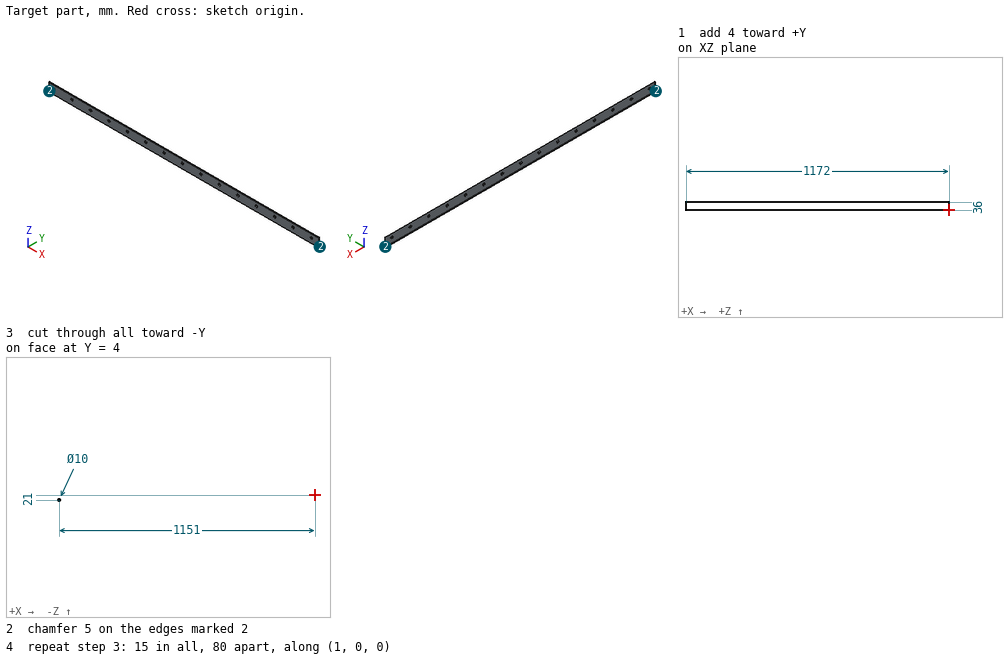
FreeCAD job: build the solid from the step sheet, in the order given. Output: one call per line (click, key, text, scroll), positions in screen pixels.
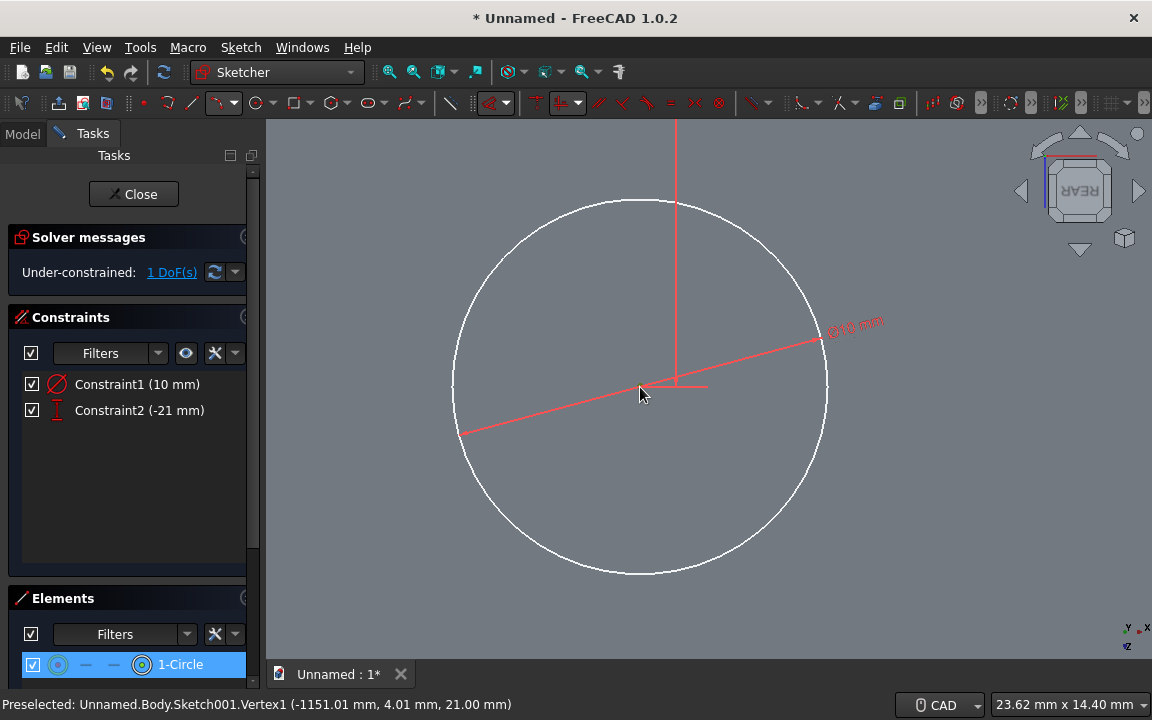
key(l)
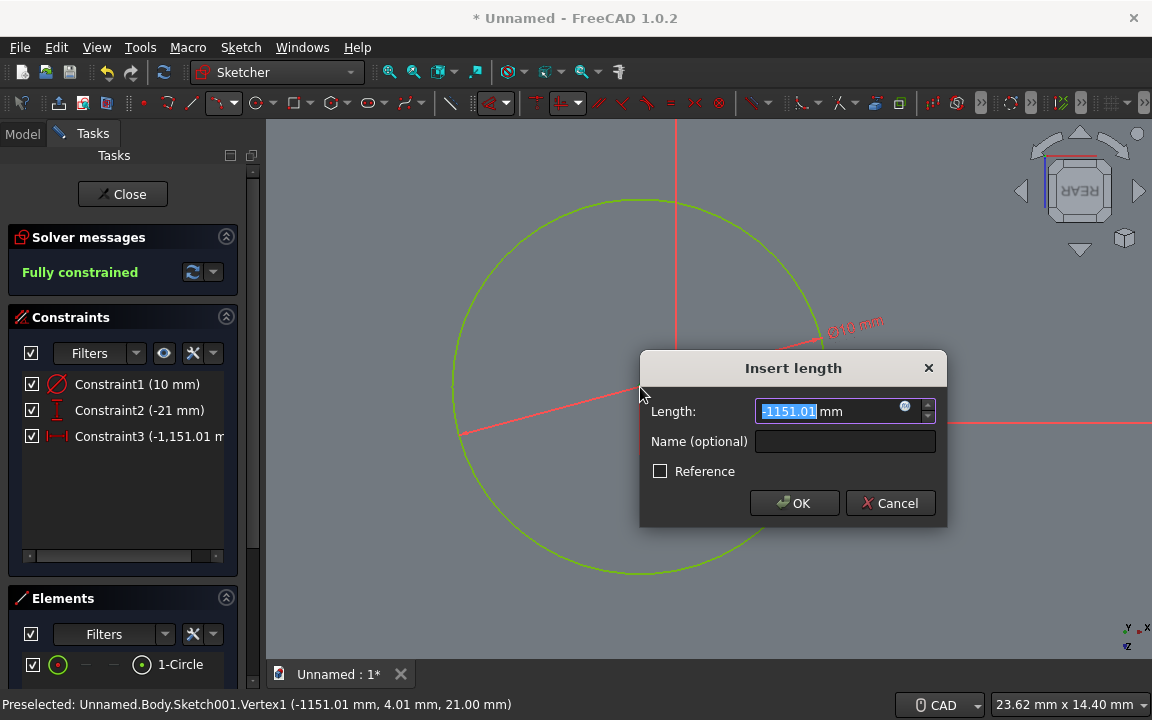
text(-1151)
key(Return)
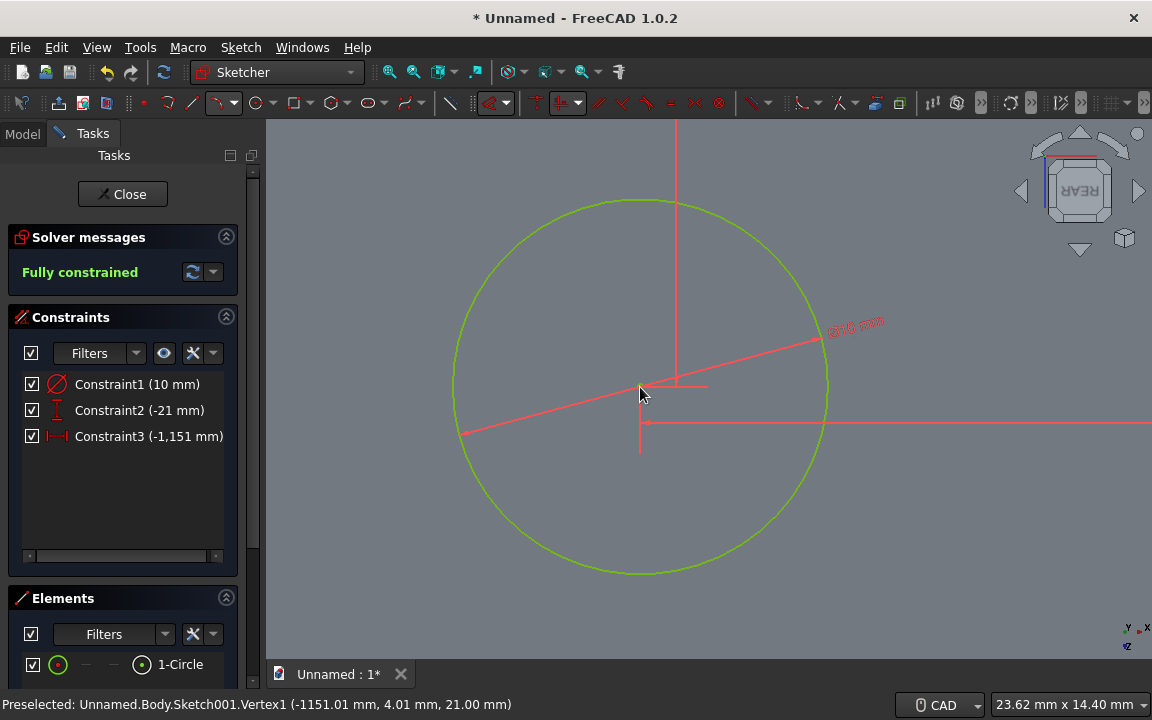
click(123, 194)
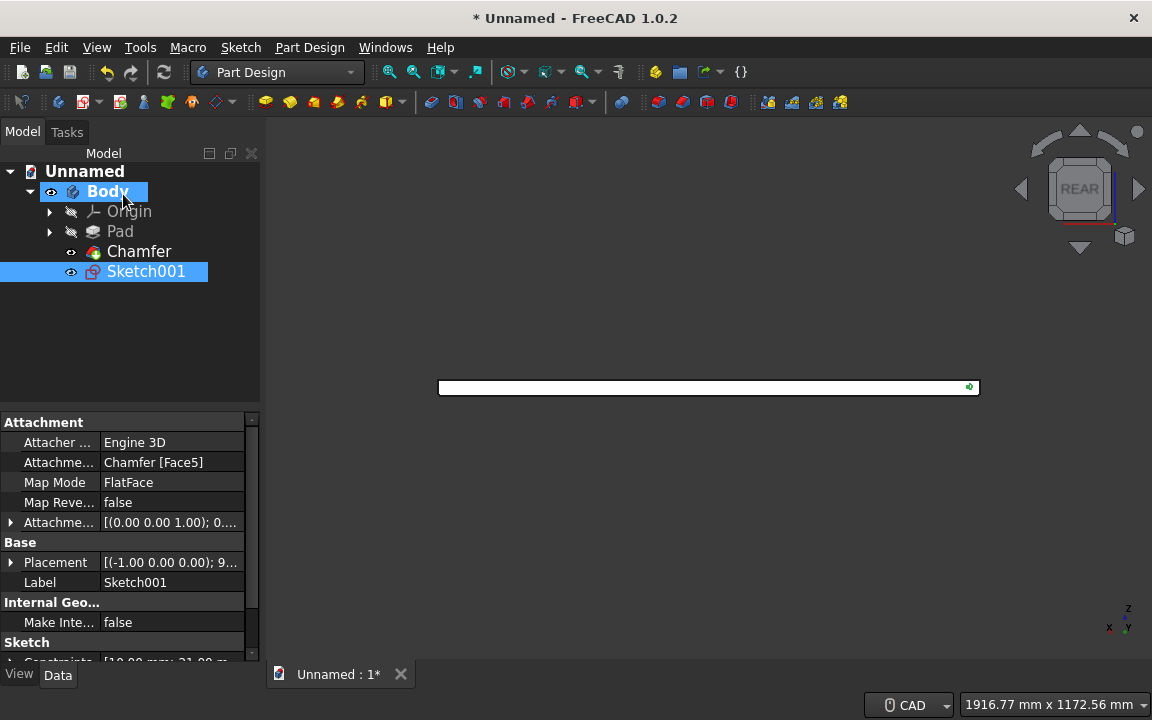
click(432, 102)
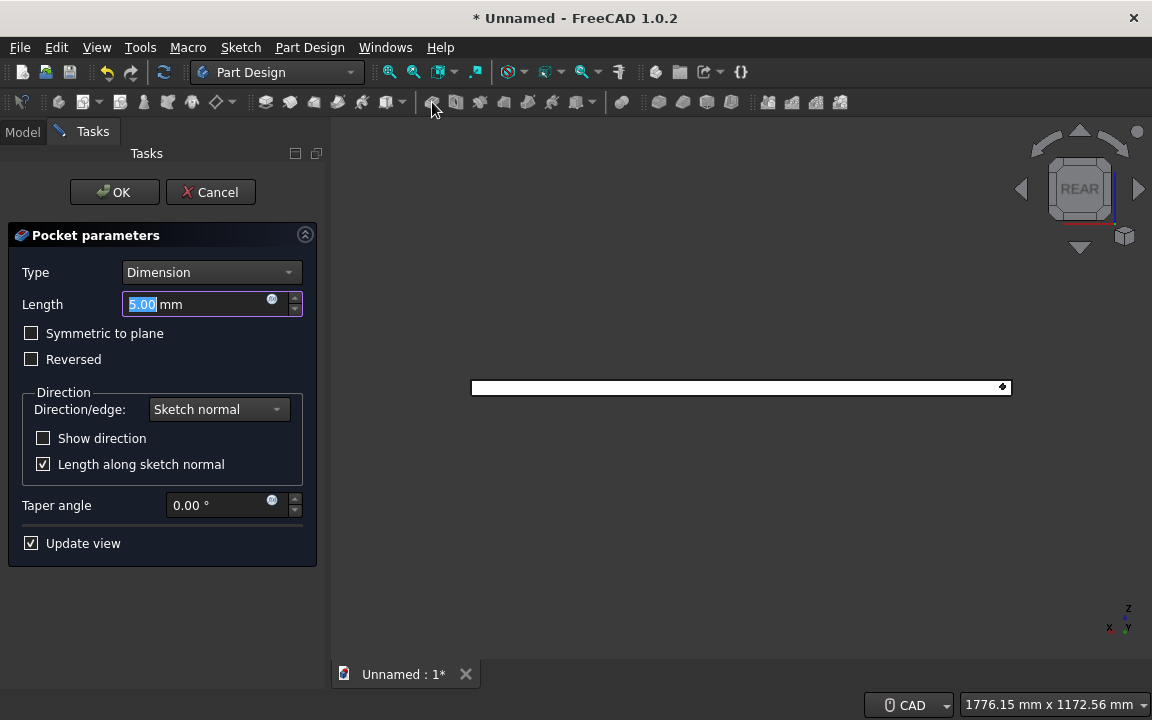
click(212, 272)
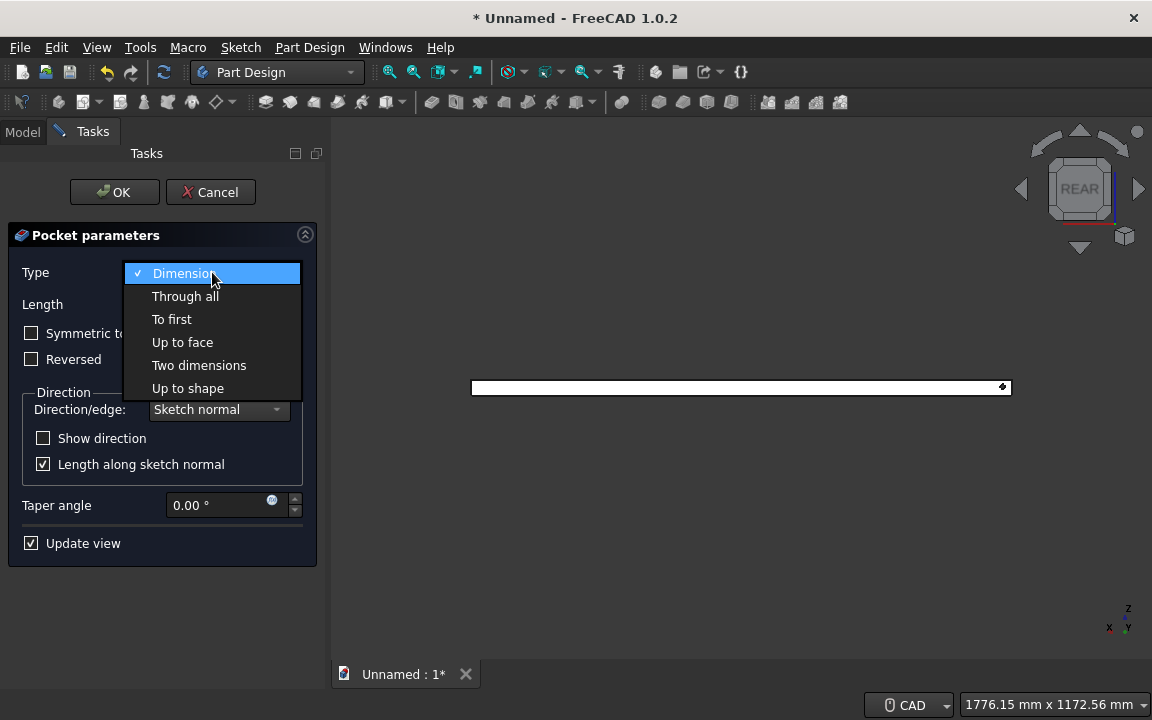
click(212, 296)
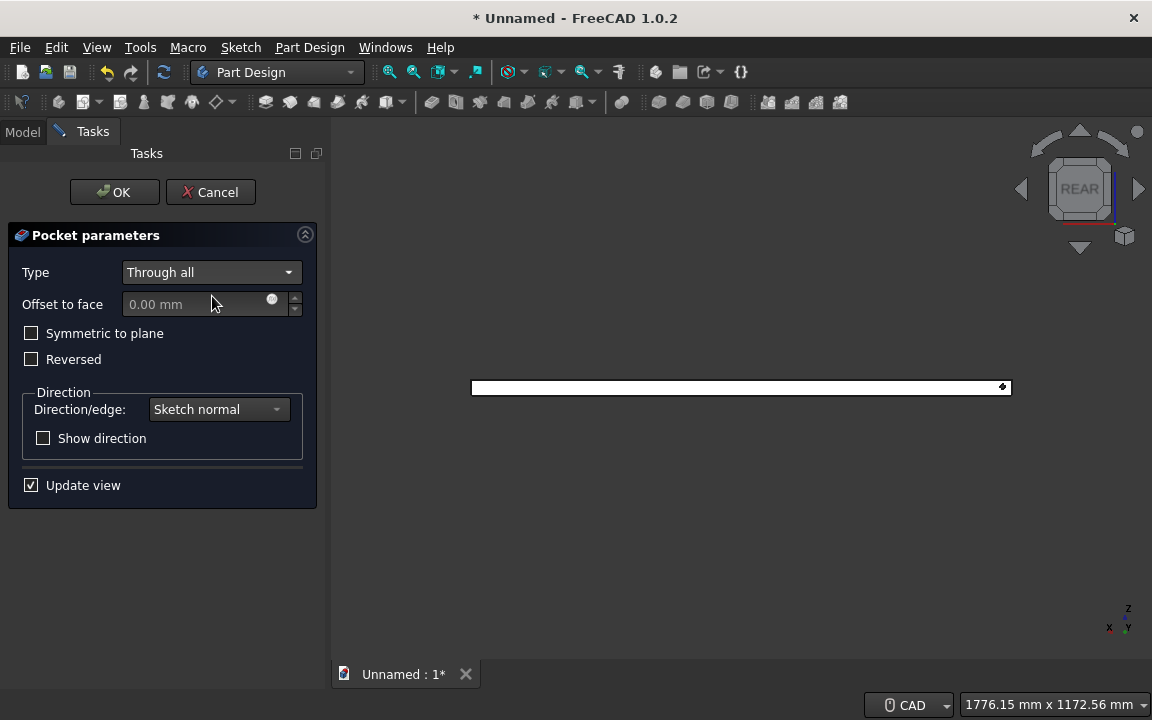
click(115, 192)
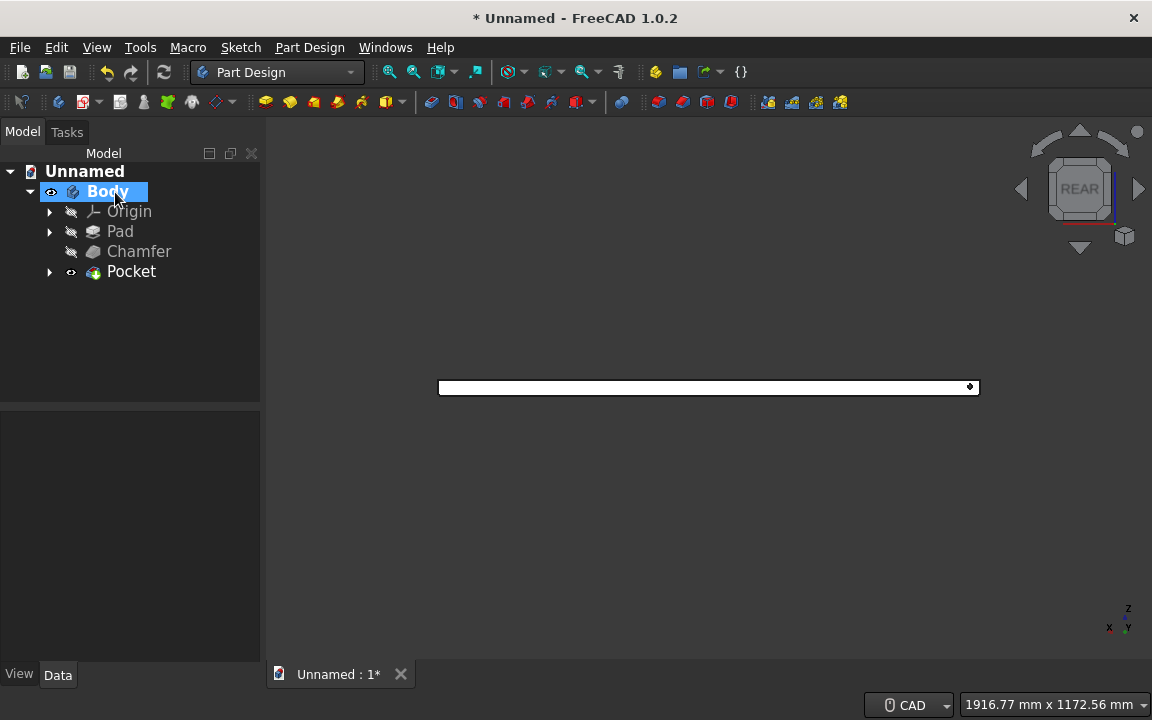
click(116, 272)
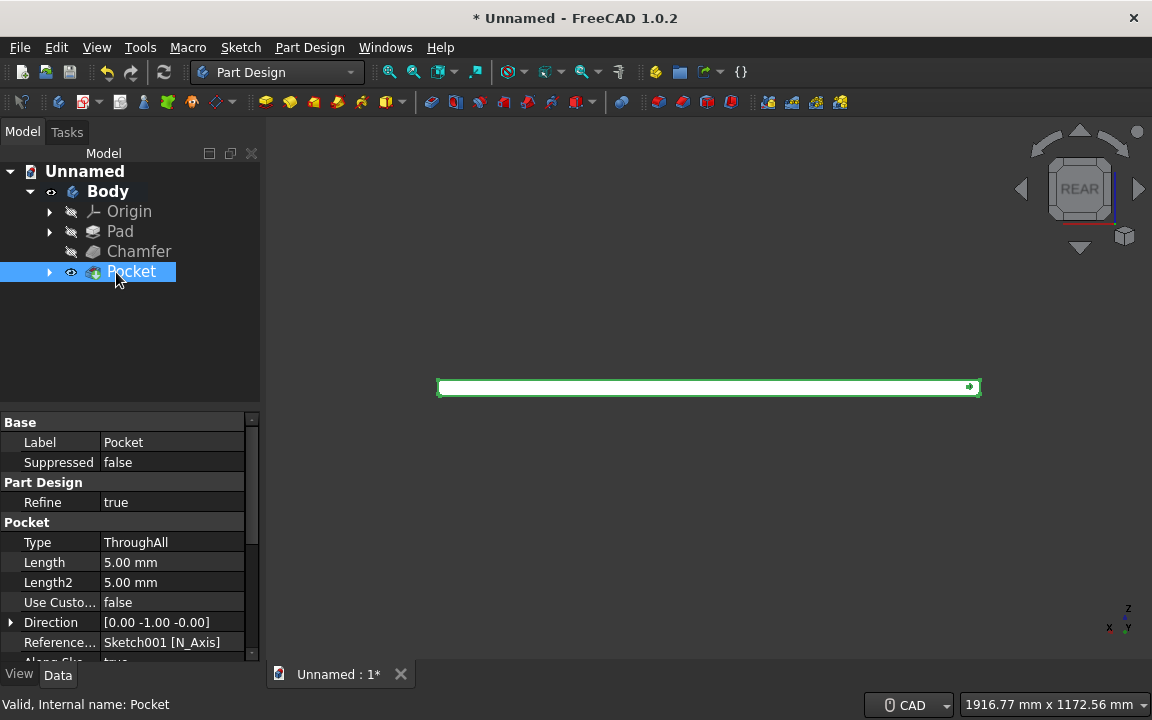
click(792, 102)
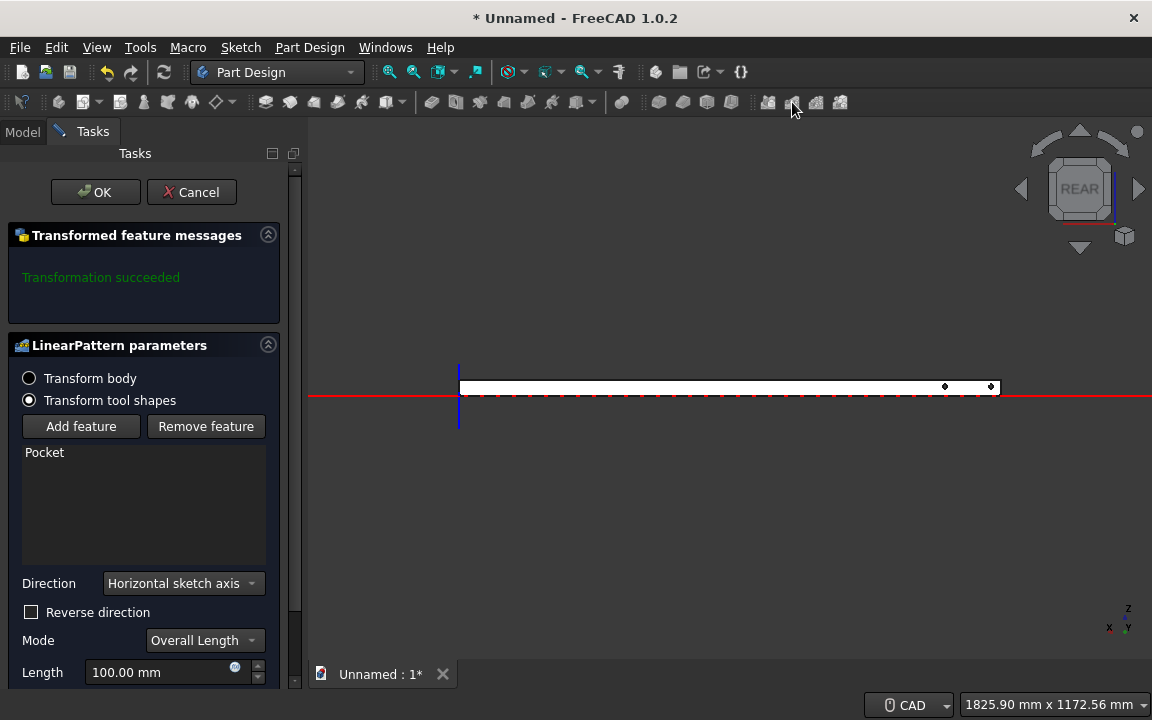
click(184, 584)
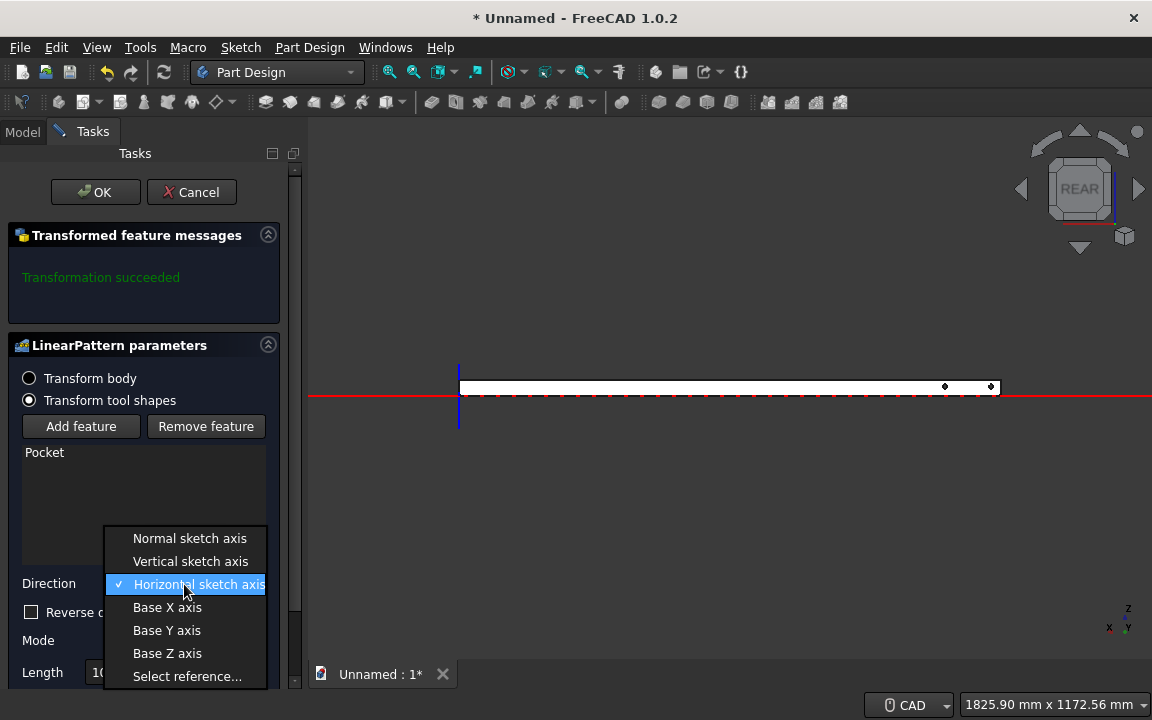
click(184, 608)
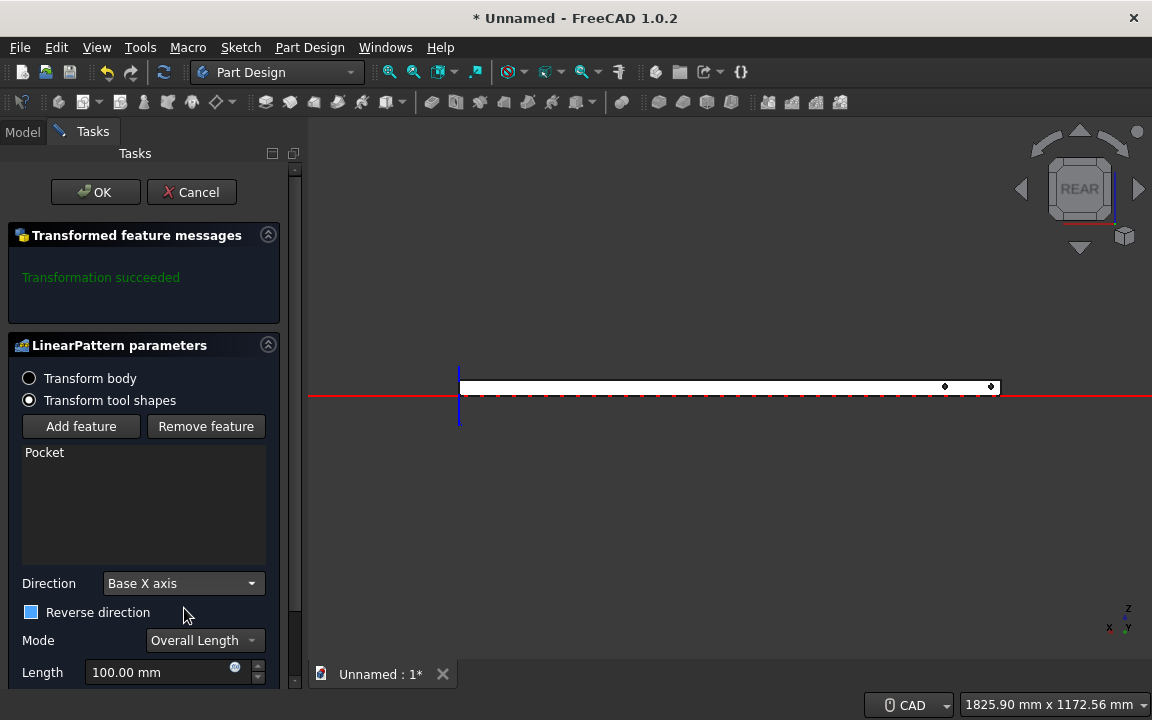
click(206, 640)